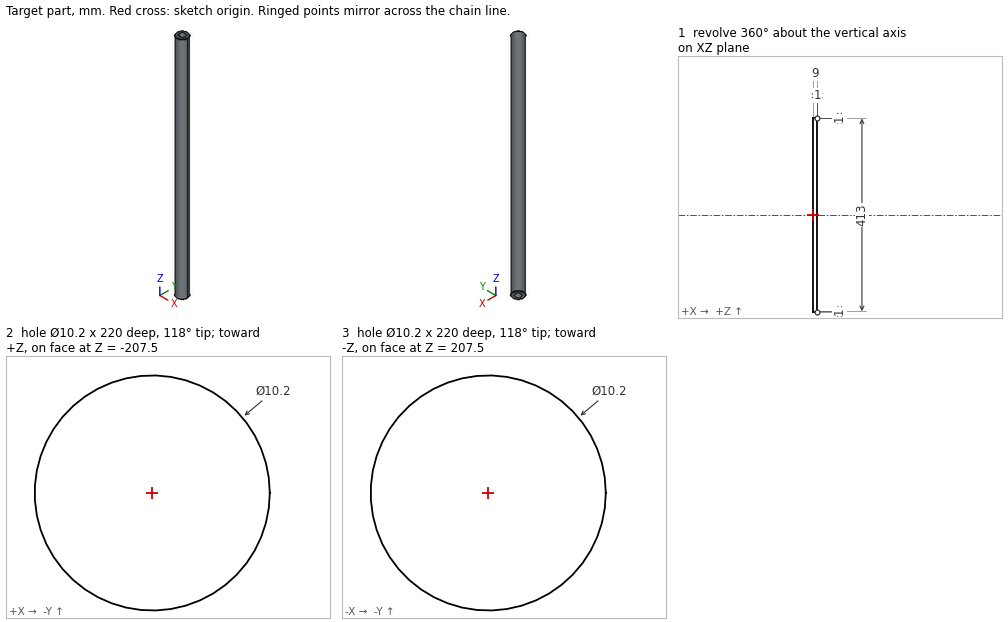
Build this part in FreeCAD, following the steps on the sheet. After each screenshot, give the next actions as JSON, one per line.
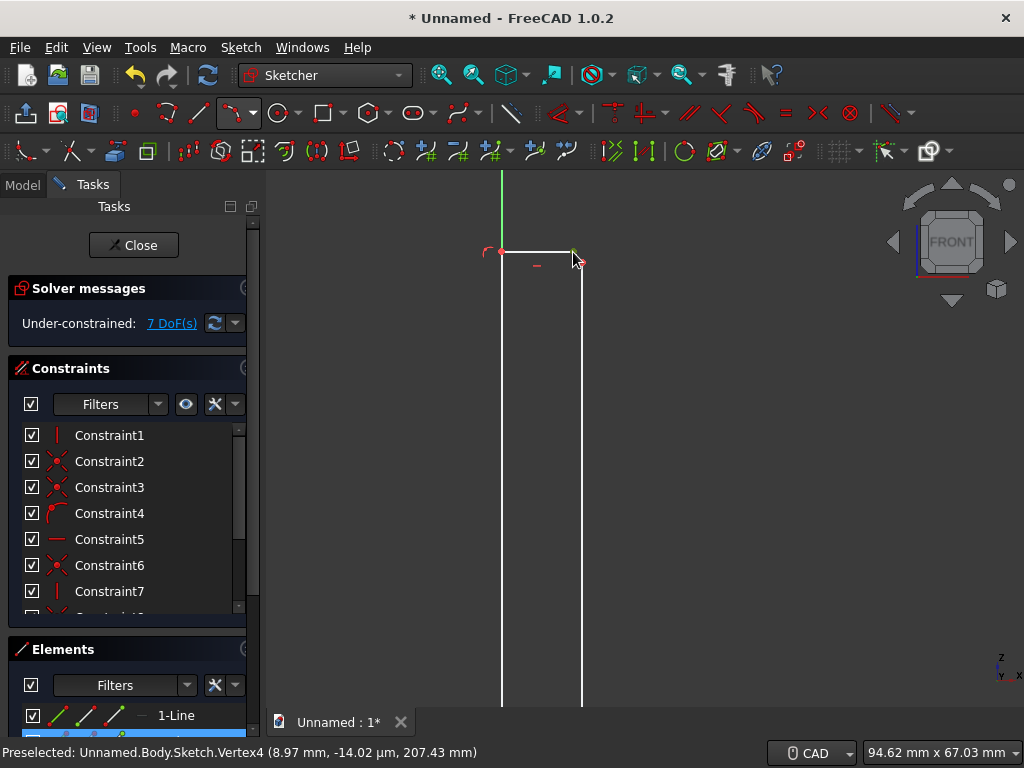
{"action": "scroll", "coordinate": [581, 255], "scroll_direction": "down", "scroll_amount": 11}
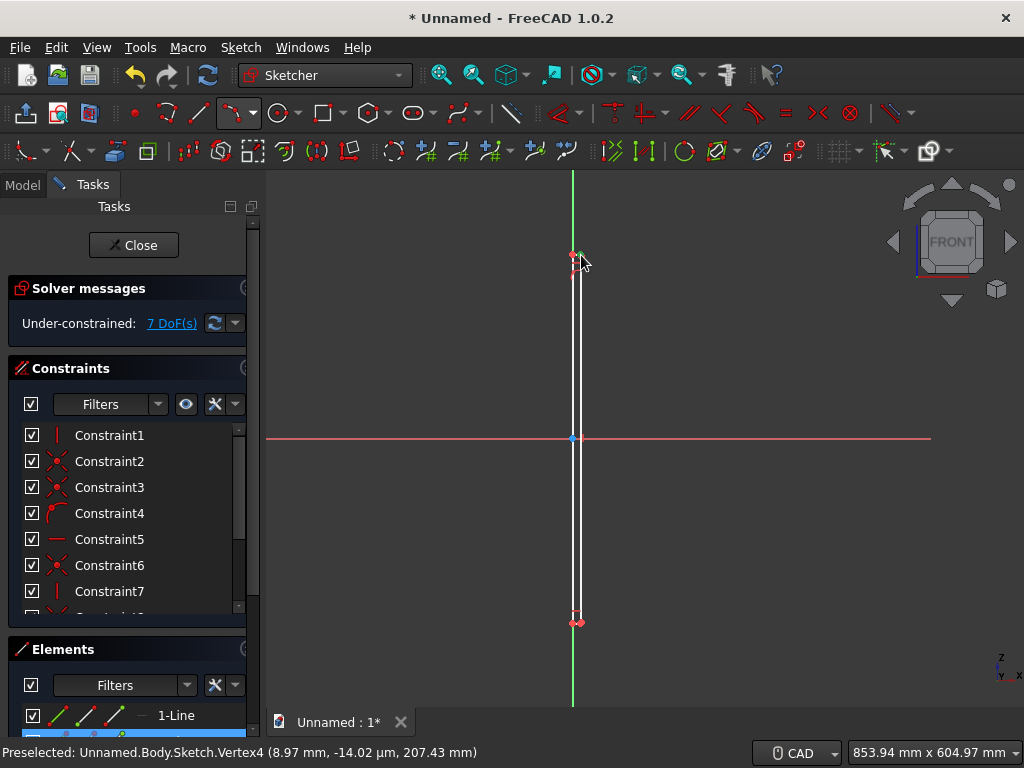
{"action": "scroll", "coordinate": [581, 624], "scroll_direction": "up", "scroll_amount": 11}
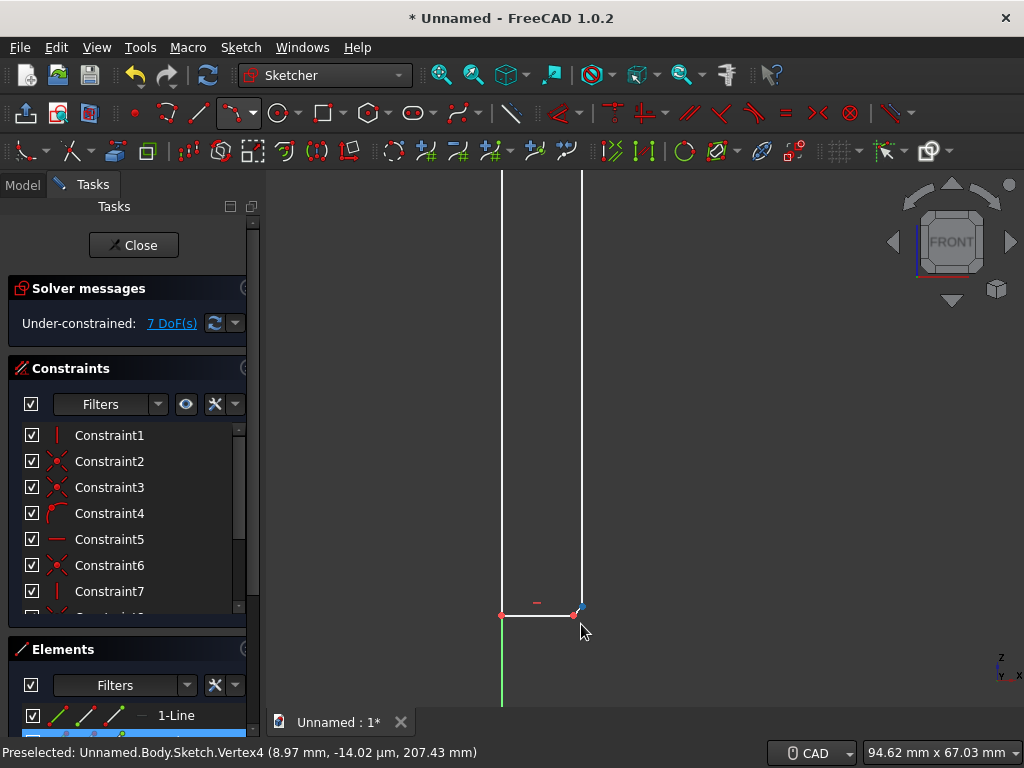
{"action": "left_click", "coordinate": [573, 616]}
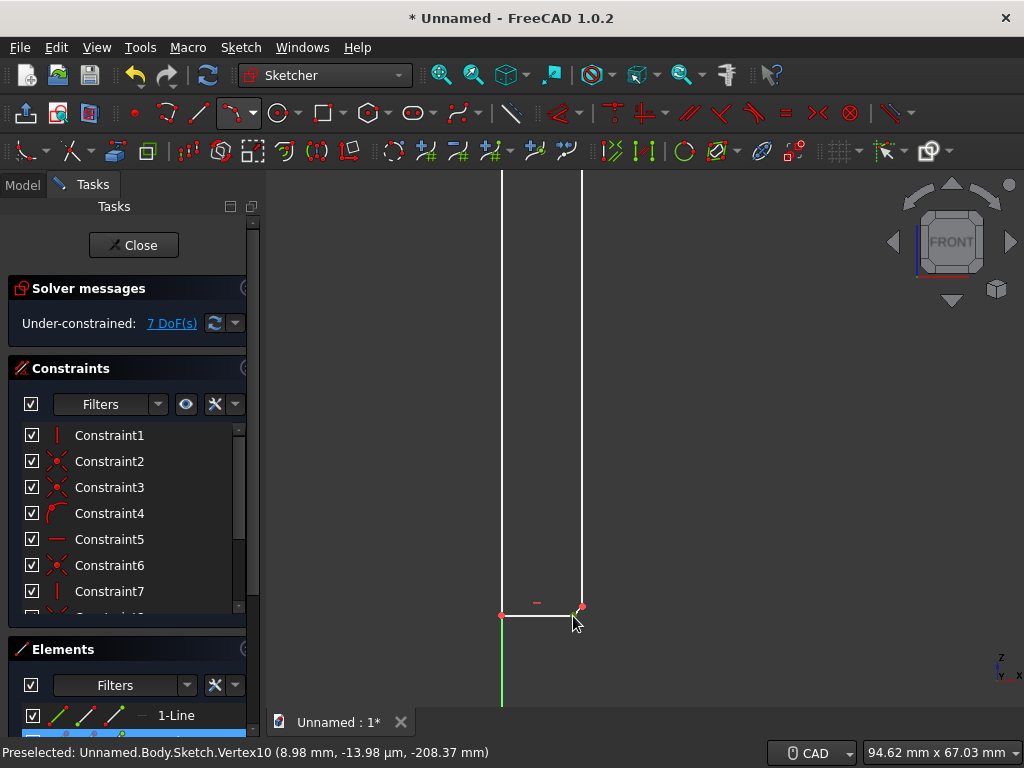
{"action": "scroll", "coordinate": [581, 624], "scroll_direction": "down", "scroll_amount": 11}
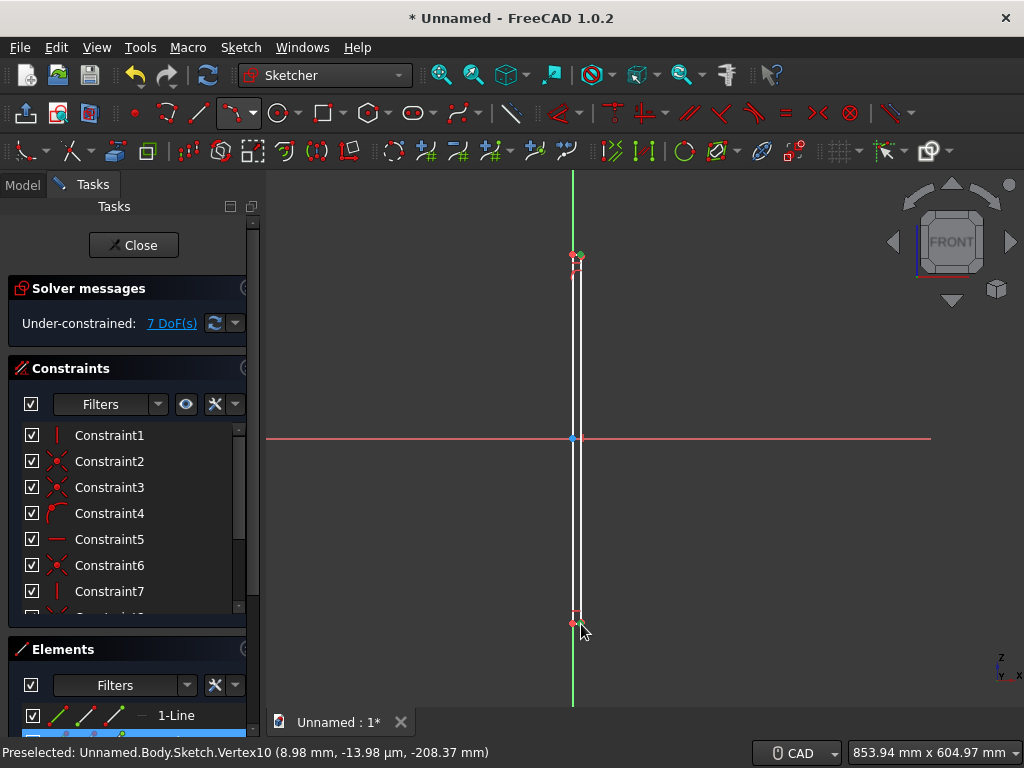
{"action": "left_click", "coordinate": [334, 439]}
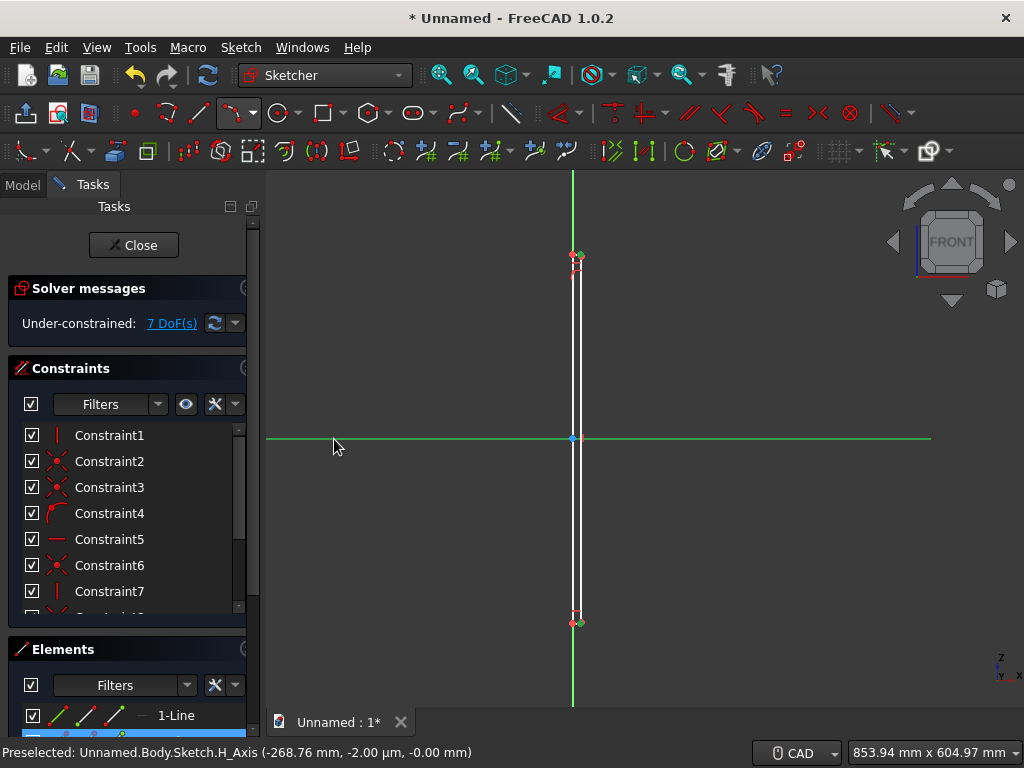
{"action": "key", "text": "s"}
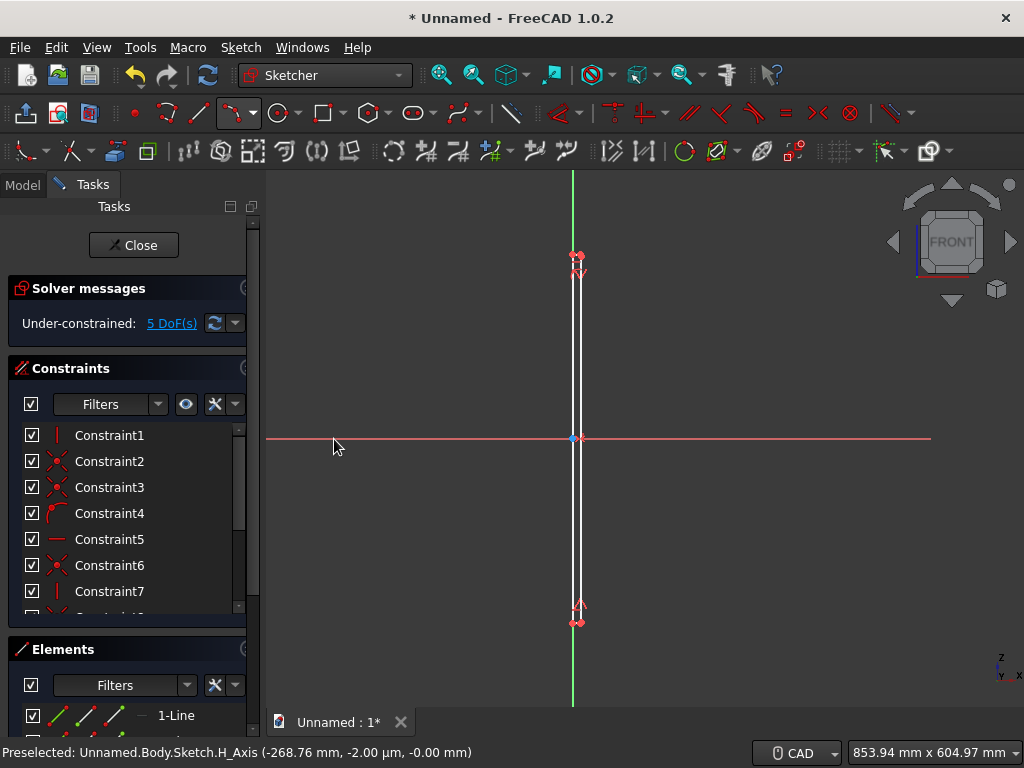
{"action": "key", "text": "d"}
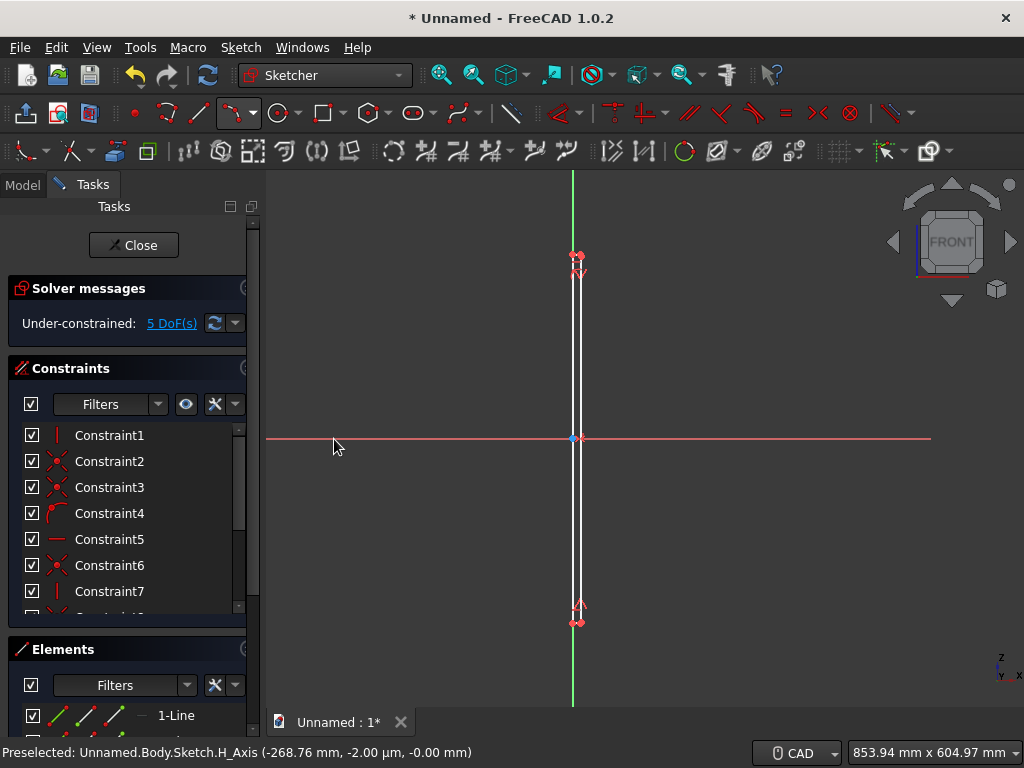
{"action": "scroll", "coordinate": [577, 255], "scroll_direction": "up", "scroll_amount": 9}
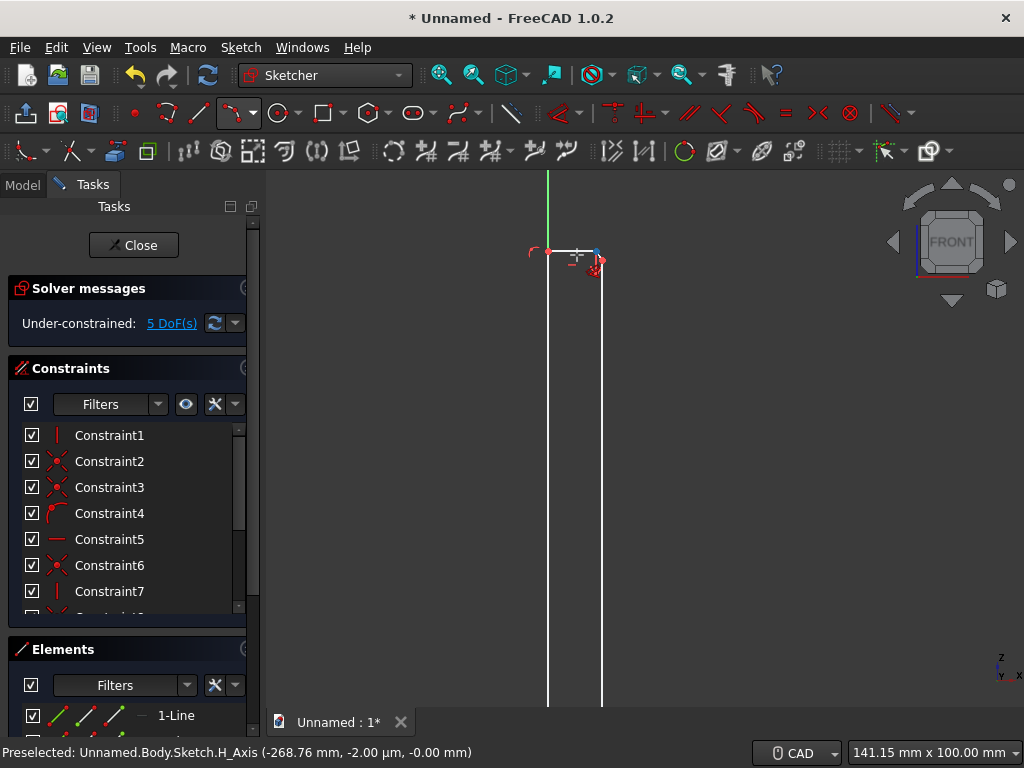
{"action": "left_click", "coordinate": [572, 251]}
{"action": "left_click", "coordinate": [572, 217]}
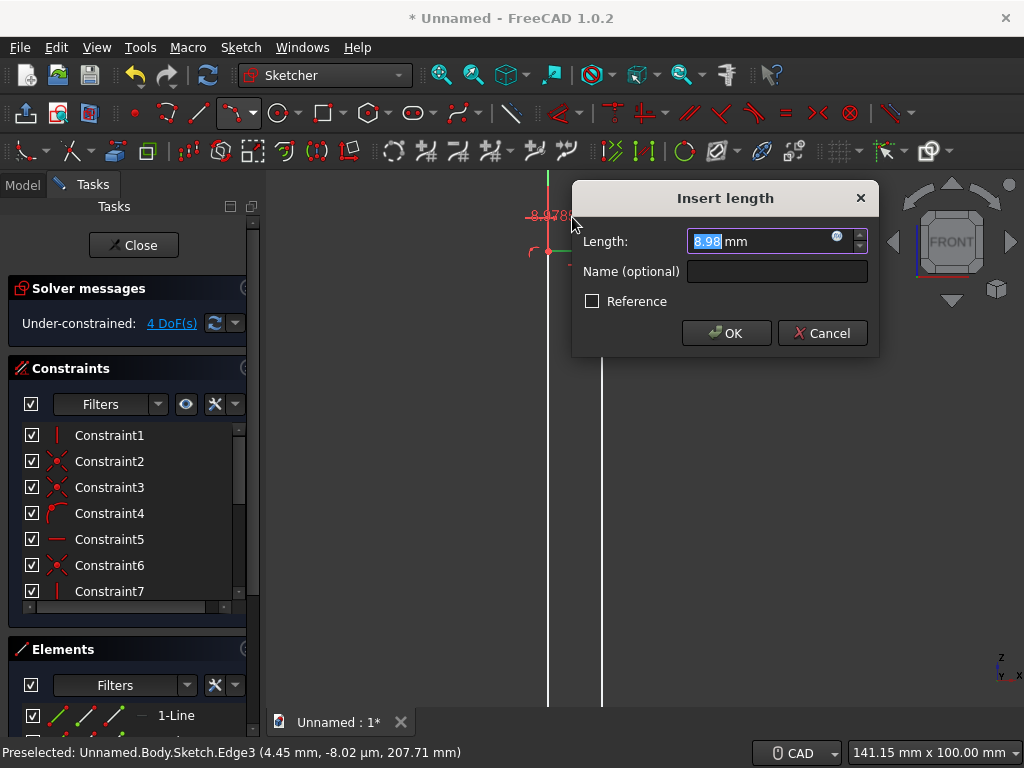
{"action": "type", "text": "9"}
{"action": "key", "text": "Return"}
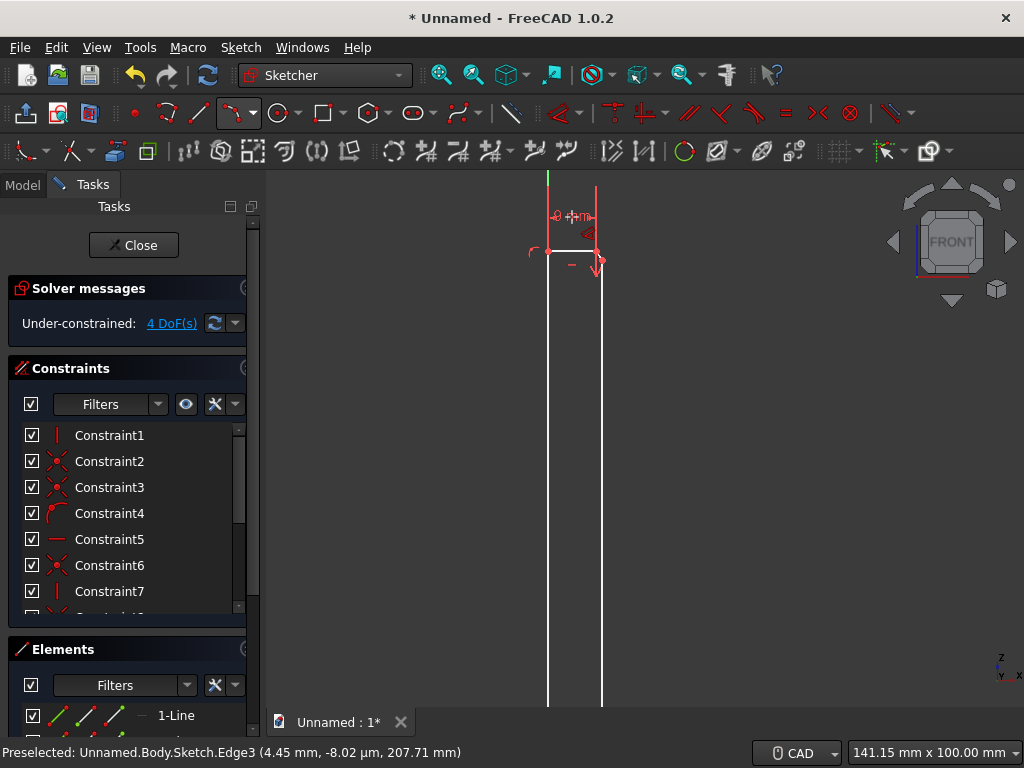
{"action": "scroll", "coordinate": [599, 256], "scroll_direction": "up", "scroll_amount": 11}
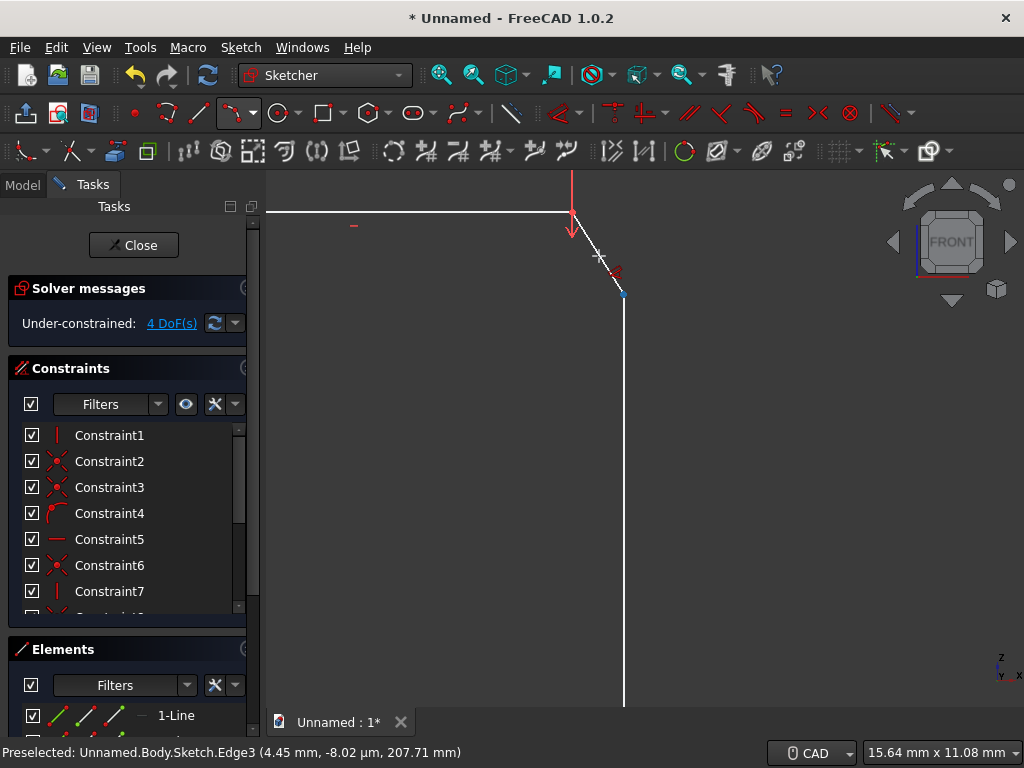
{"action": "left_click", "coordinate": [598, 253]}
{"action": "left_click", "coordinate": [598, 328]}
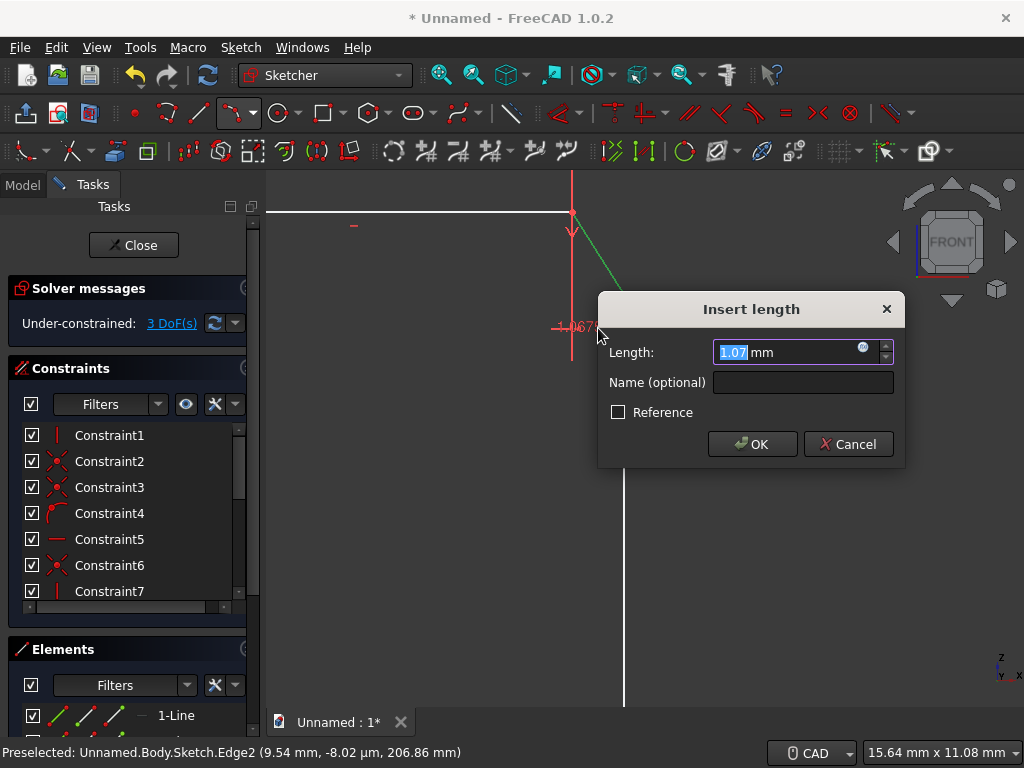
{"action": "type", "text": "1"}
{"action": "key", "text": "Return"}